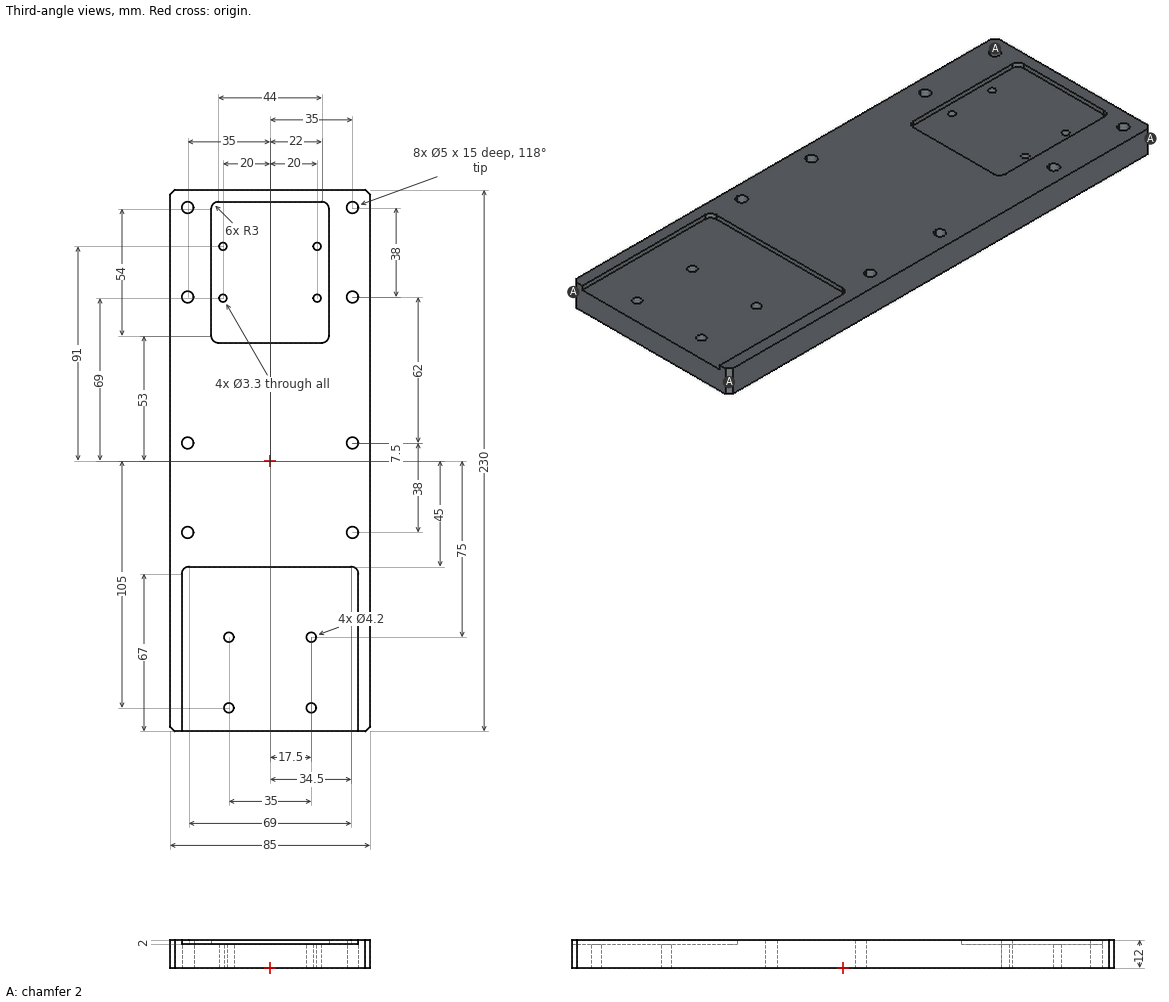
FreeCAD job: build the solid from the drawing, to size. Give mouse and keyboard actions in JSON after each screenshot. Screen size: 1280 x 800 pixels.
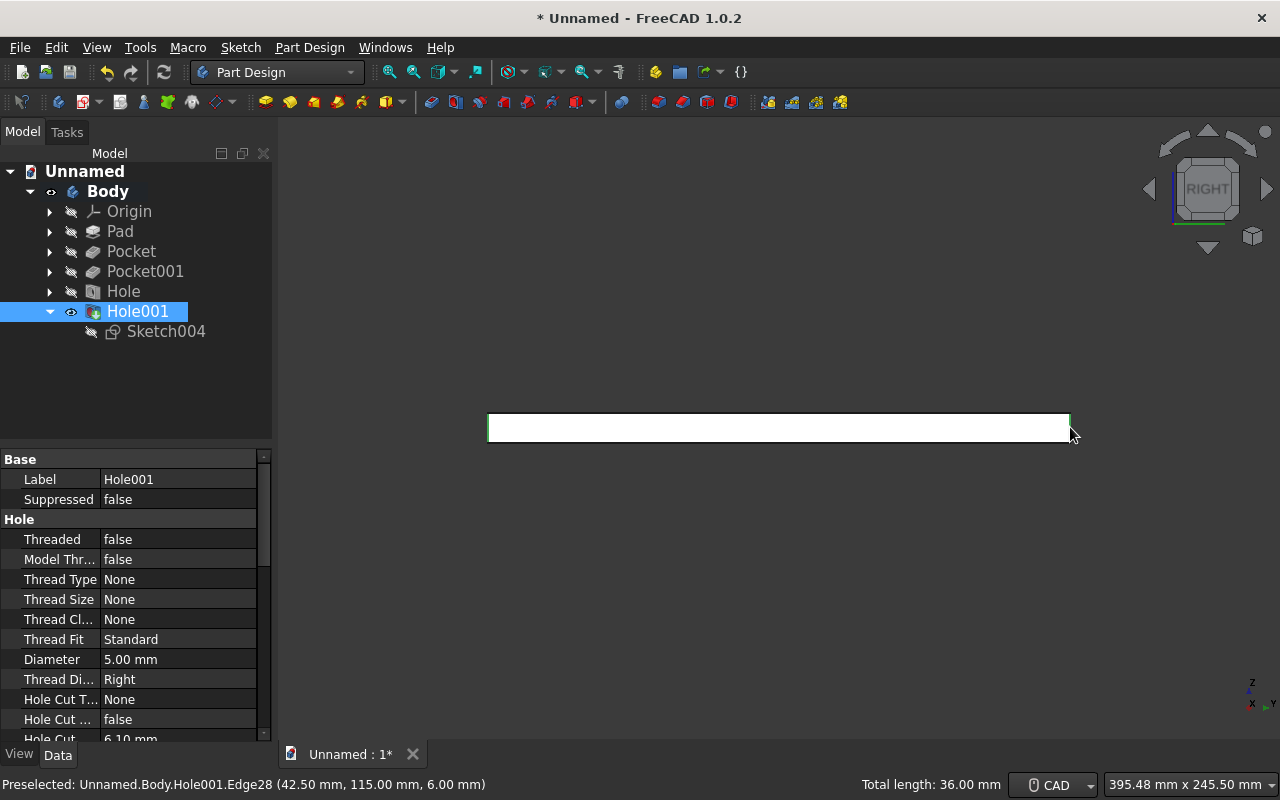
{"action": "key", "text": "5"}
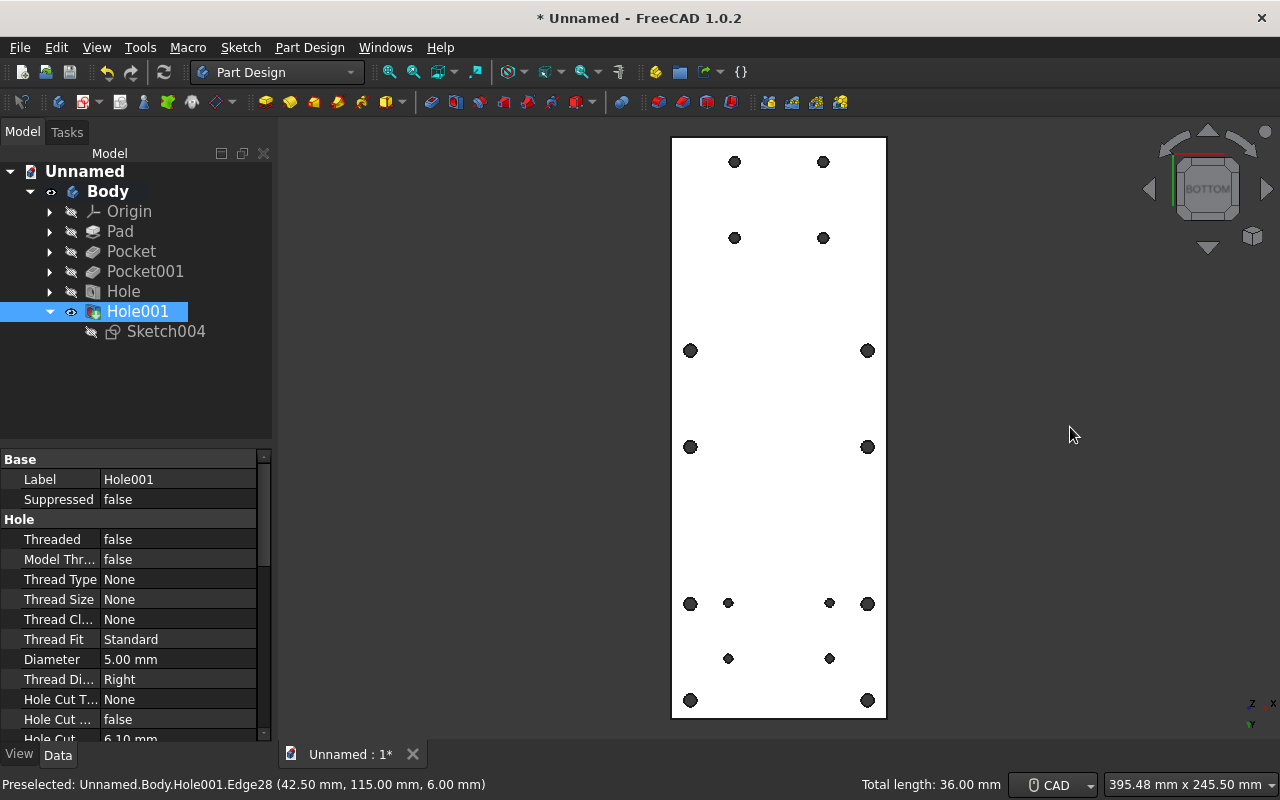
{"action": "key", "text": "4"}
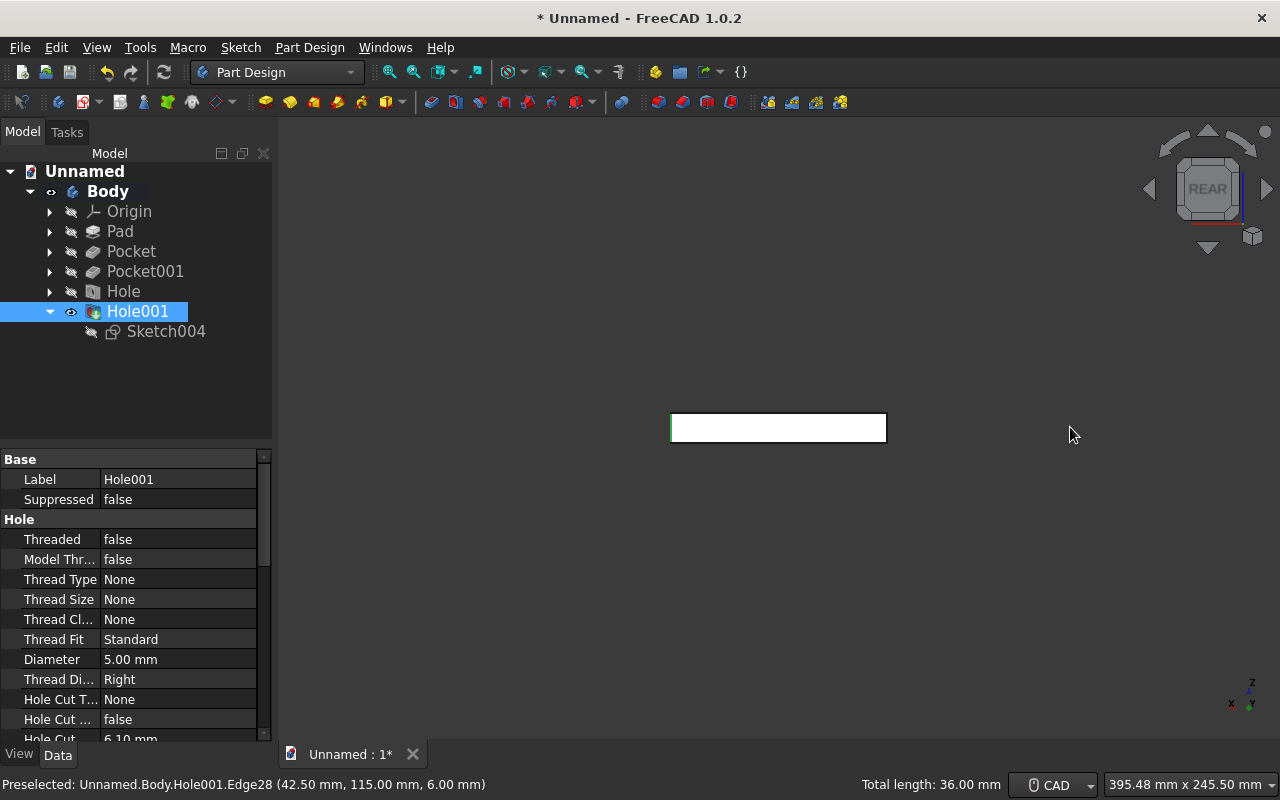
{"action": "key", "text": "v f"}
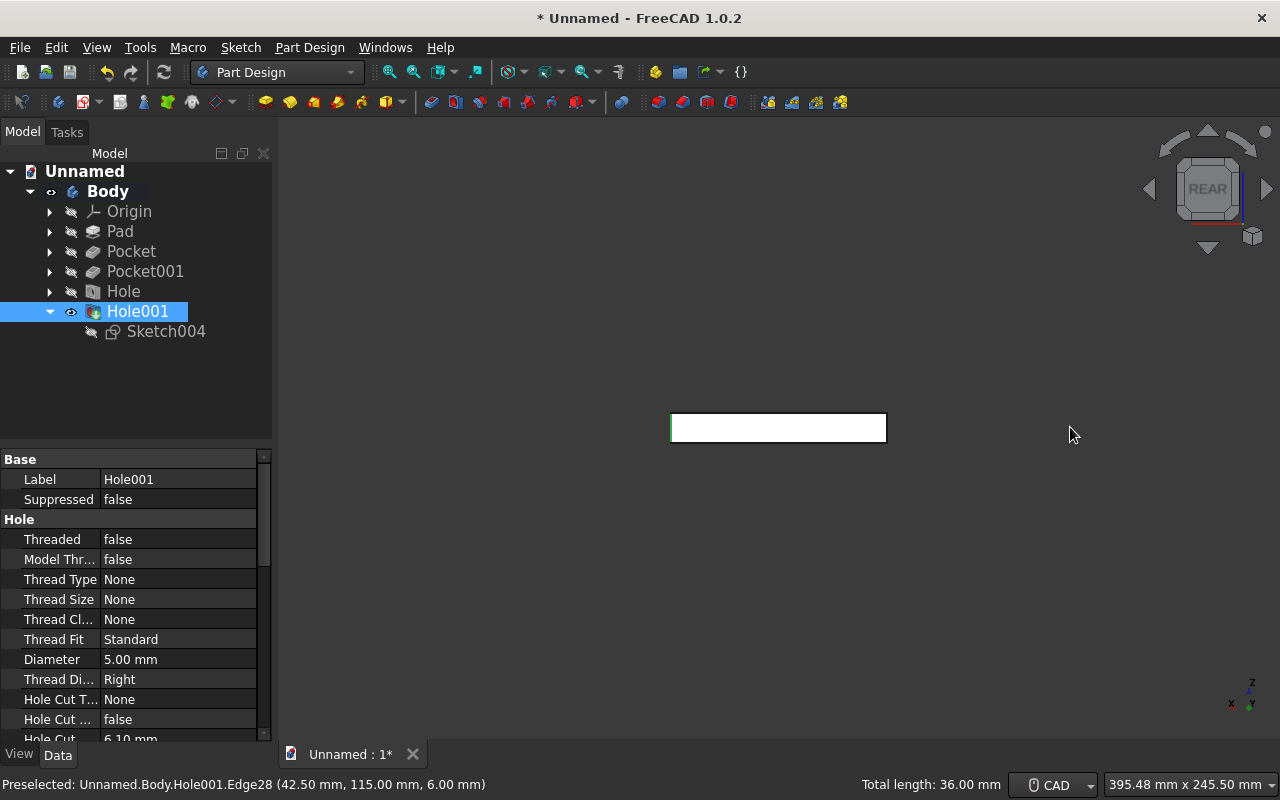
{"action": "left_click", "coordinate": [887, 427], "text": "ctrl"}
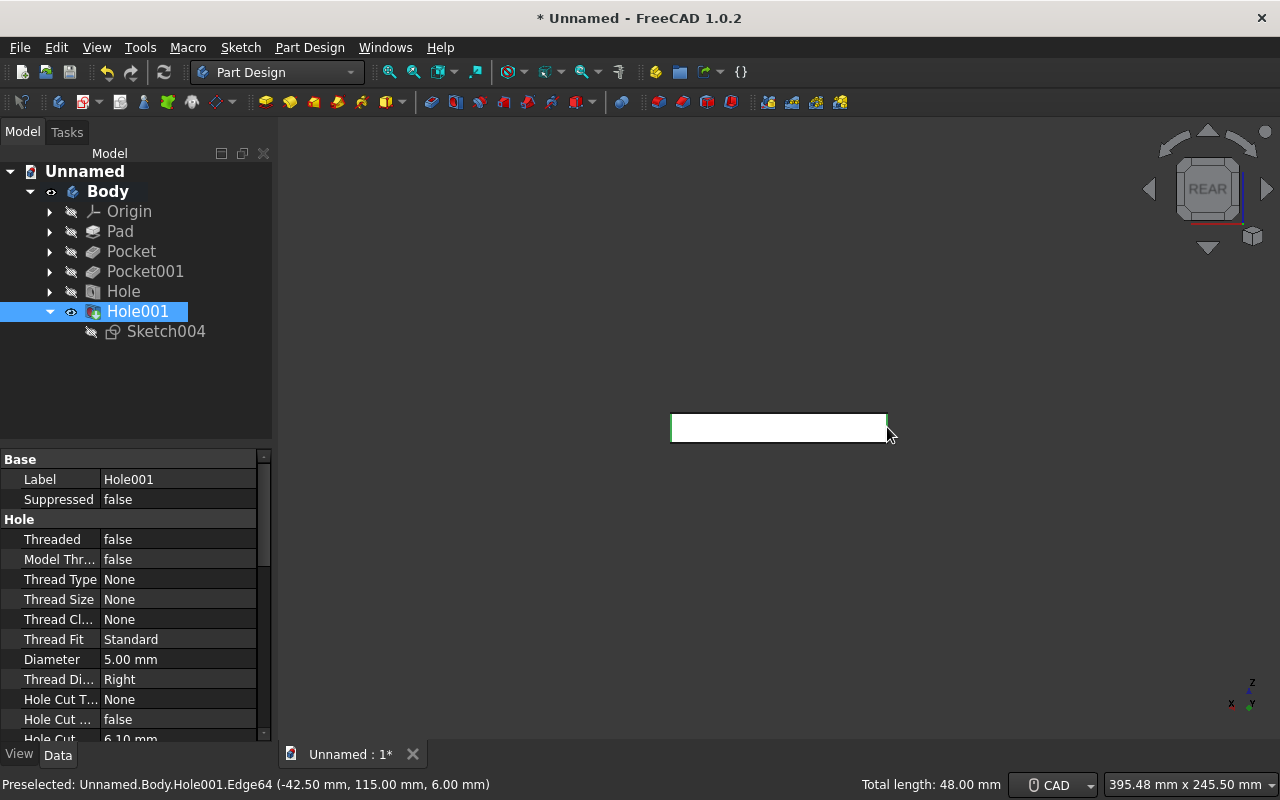
{"action": "left_click", "coordinate": [684, 102]}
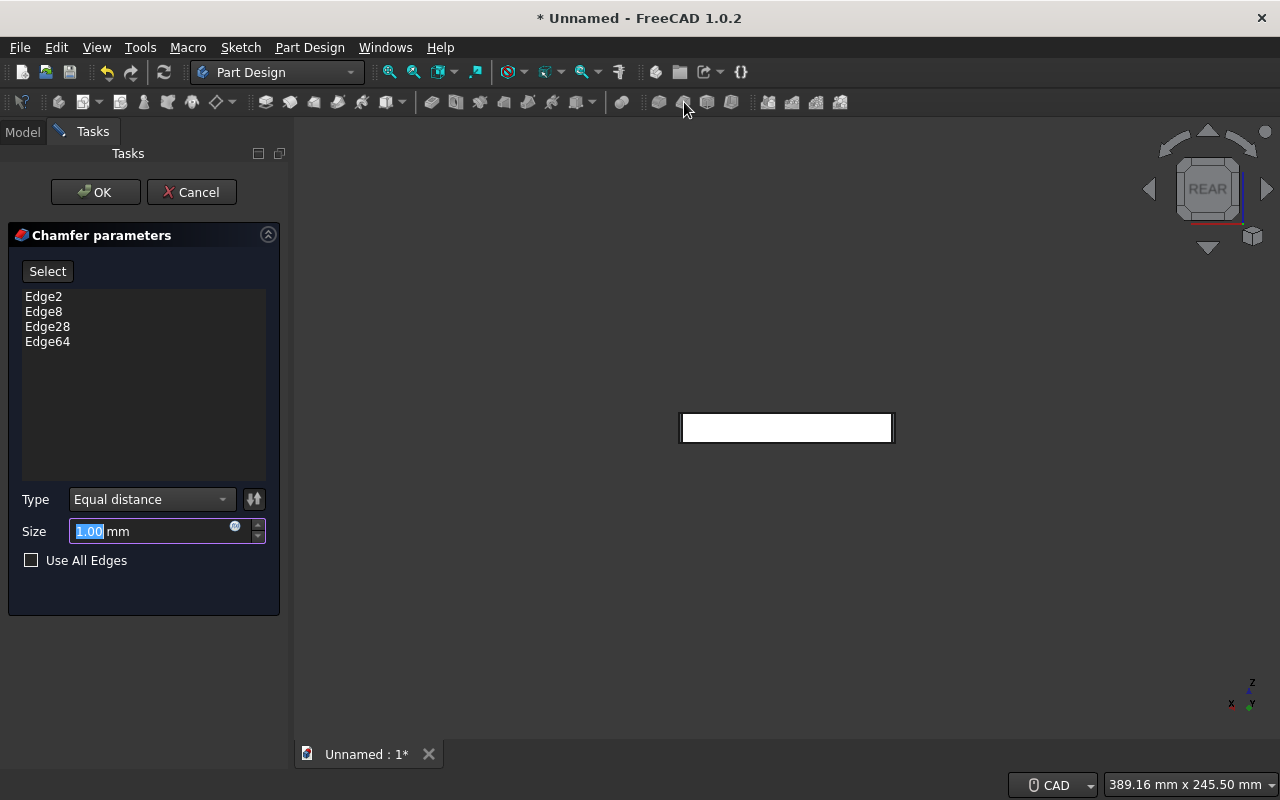
{"action": "type", "text": "2"}
{"action": "key", "text": "Tab"}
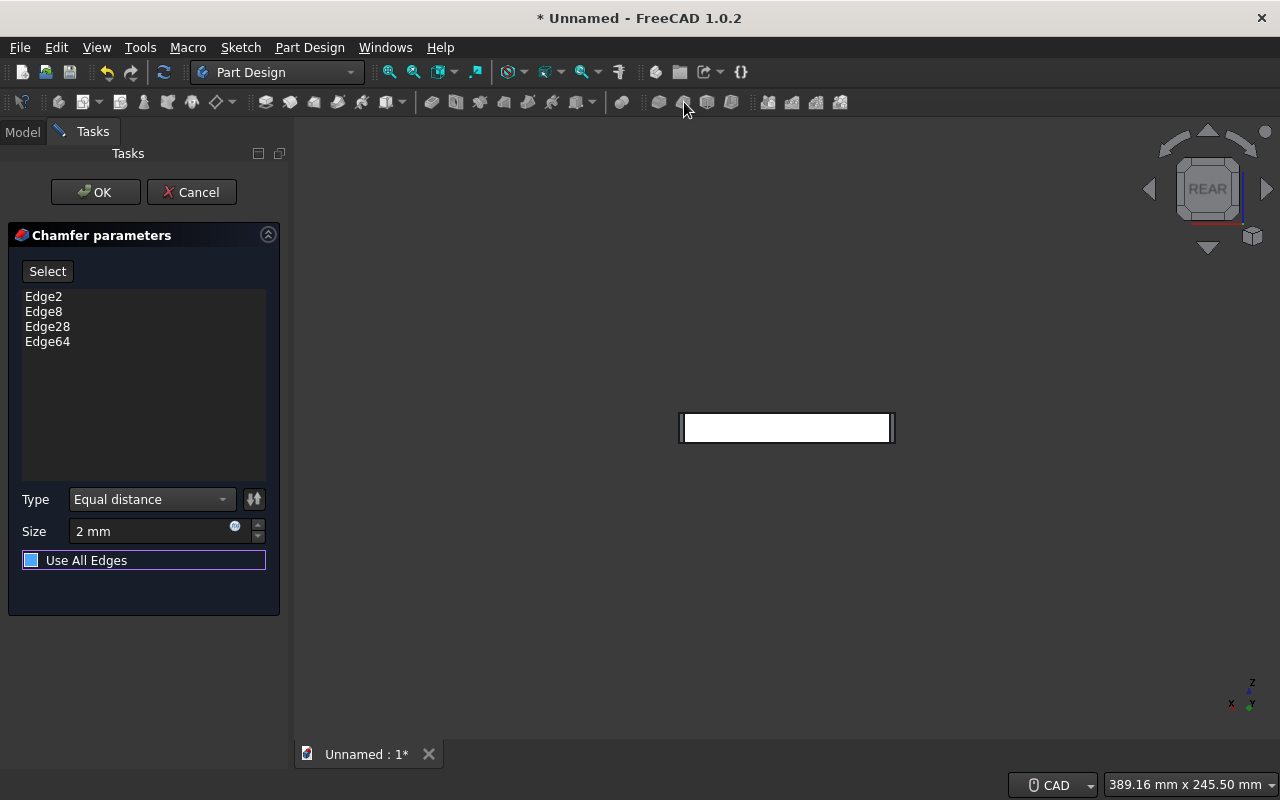
{"action": "left_click", "coordinate": [96, 192]}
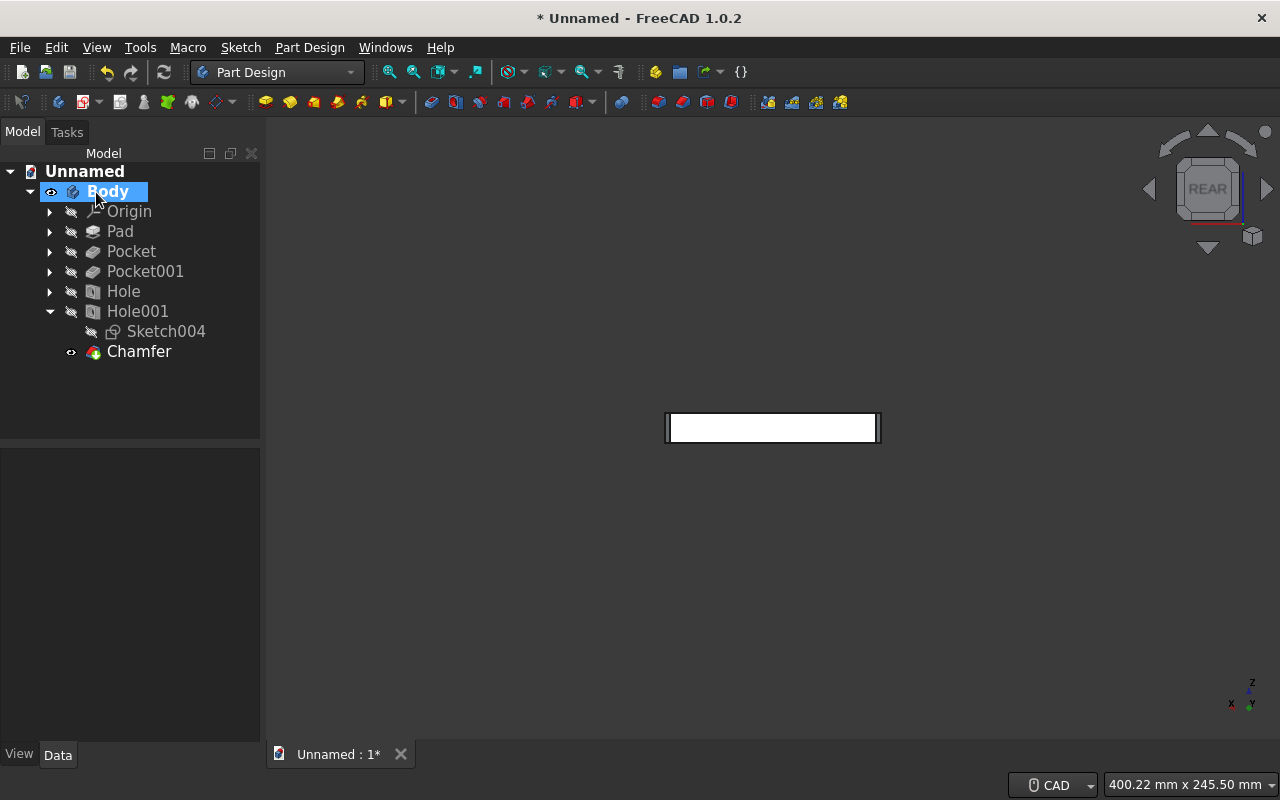
{"action": "key", "text": "0"}